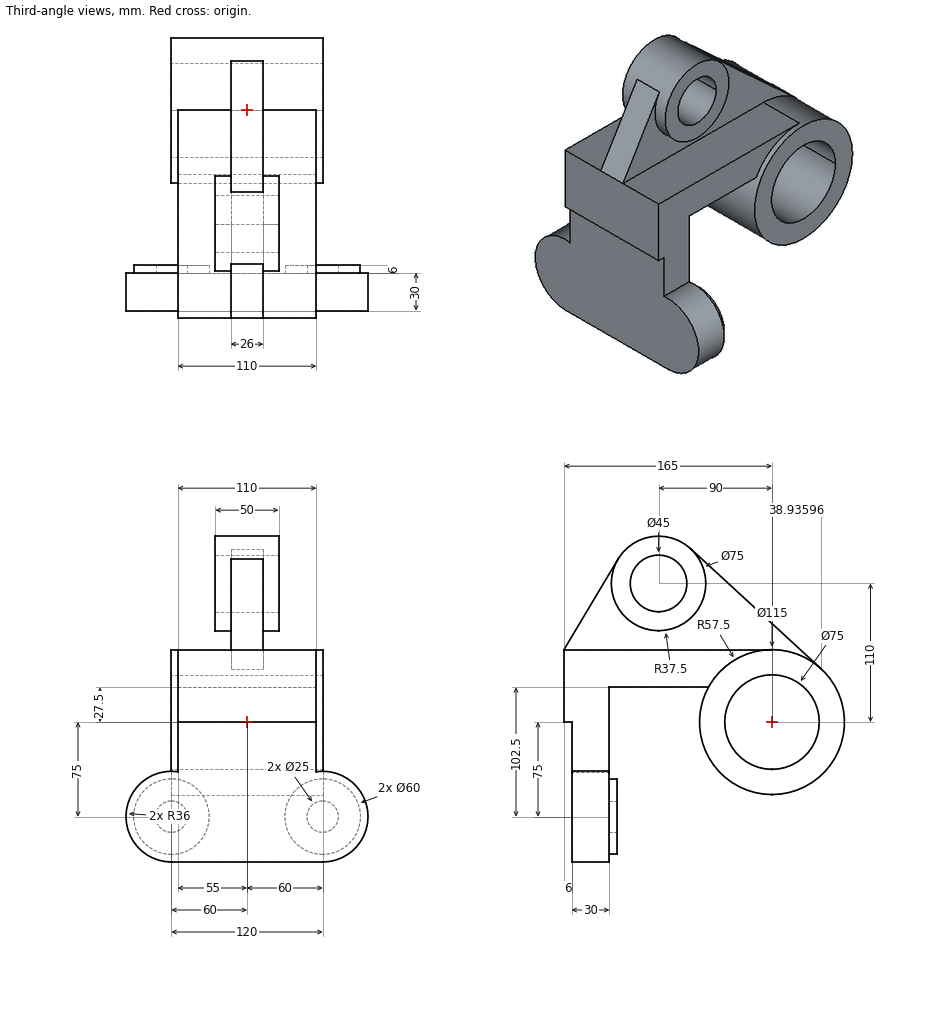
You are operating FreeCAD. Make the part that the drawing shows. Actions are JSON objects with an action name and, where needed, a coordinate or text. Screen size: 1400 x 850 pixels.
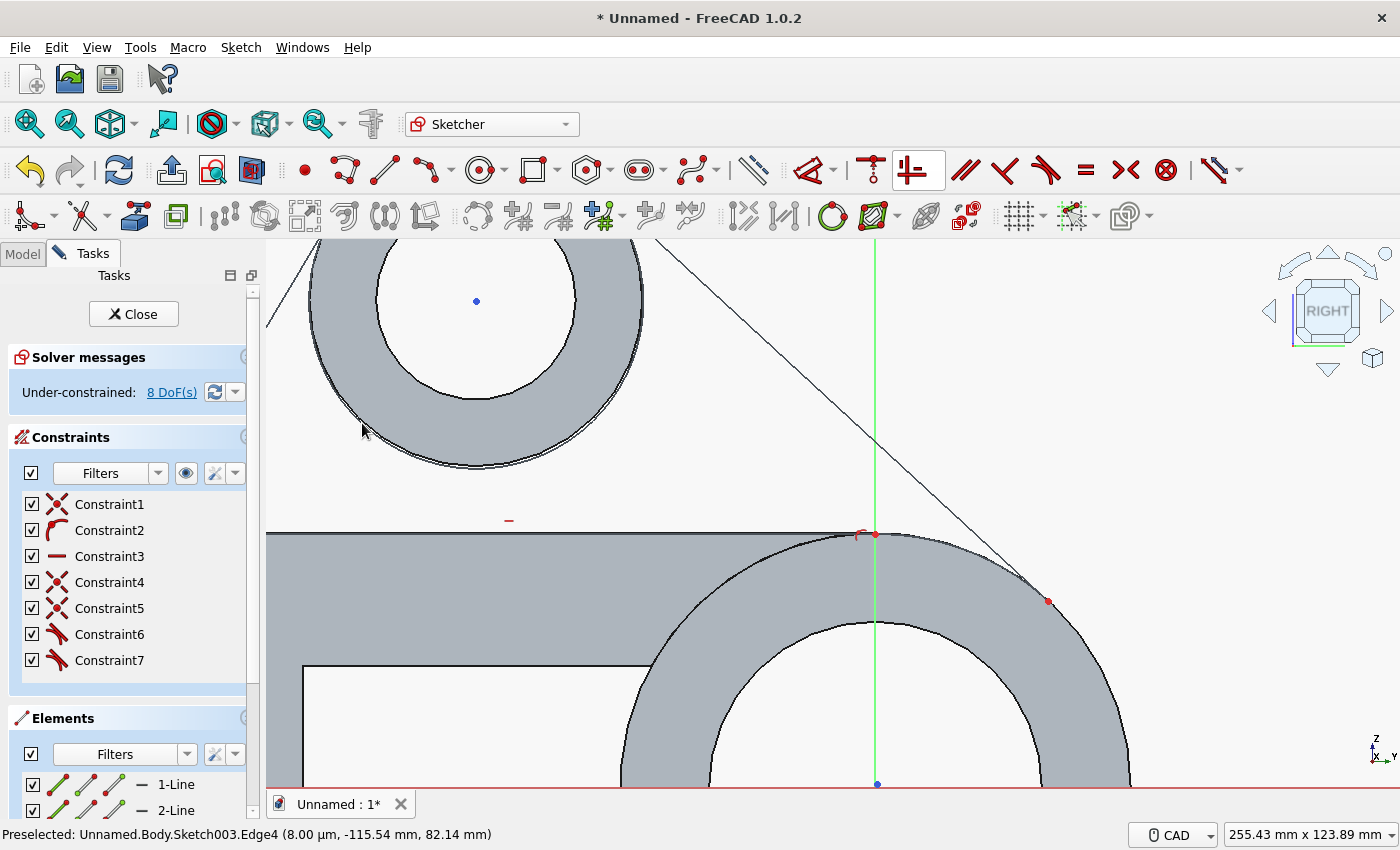
{"action": "scroll", "coordinate": [970, 552], "scroll_direction": "down", "scroll_amount": 3}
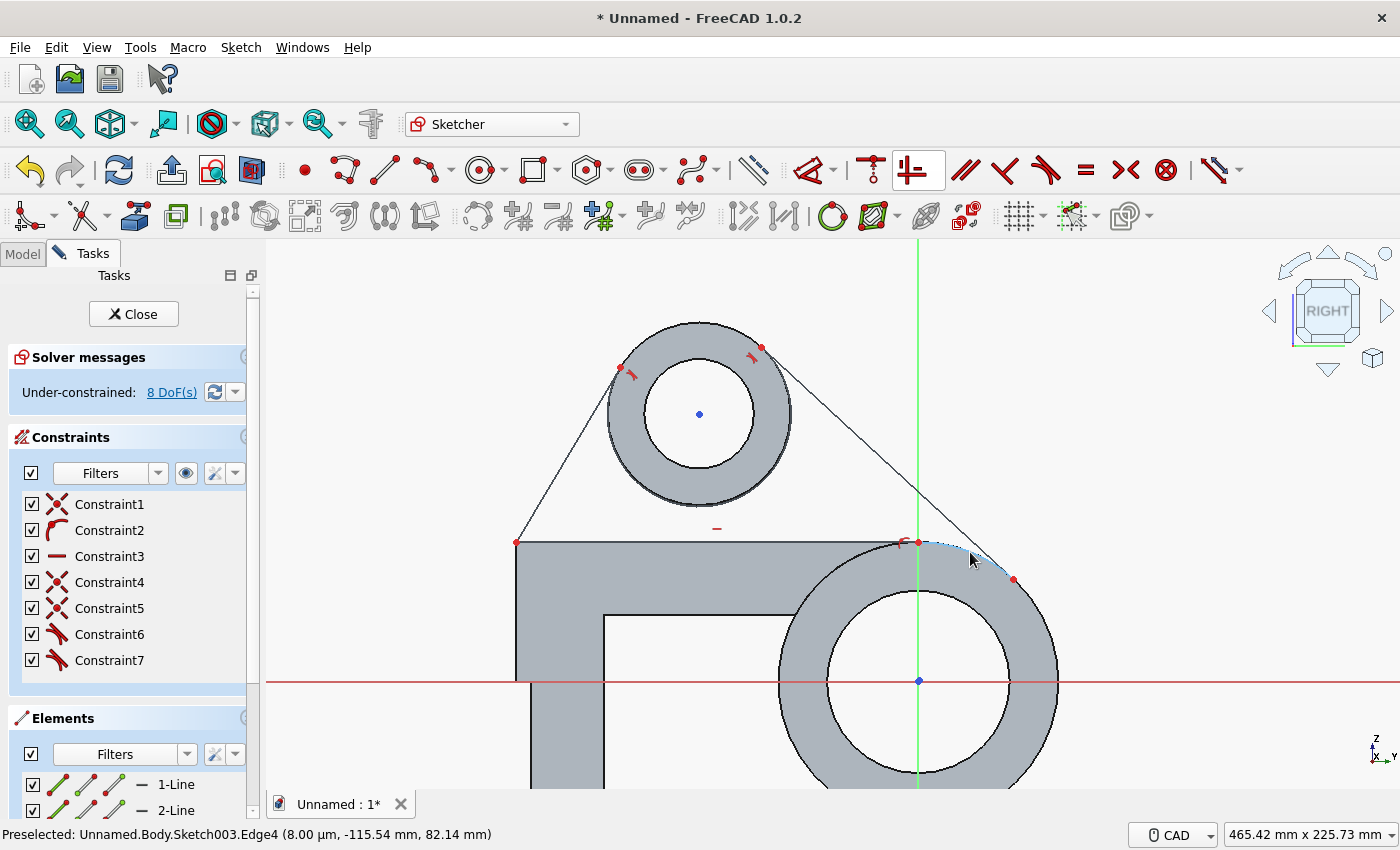
{"action": "left_click_drag", "start_coordinate": [908, 670], "coordinate": [930, 692]}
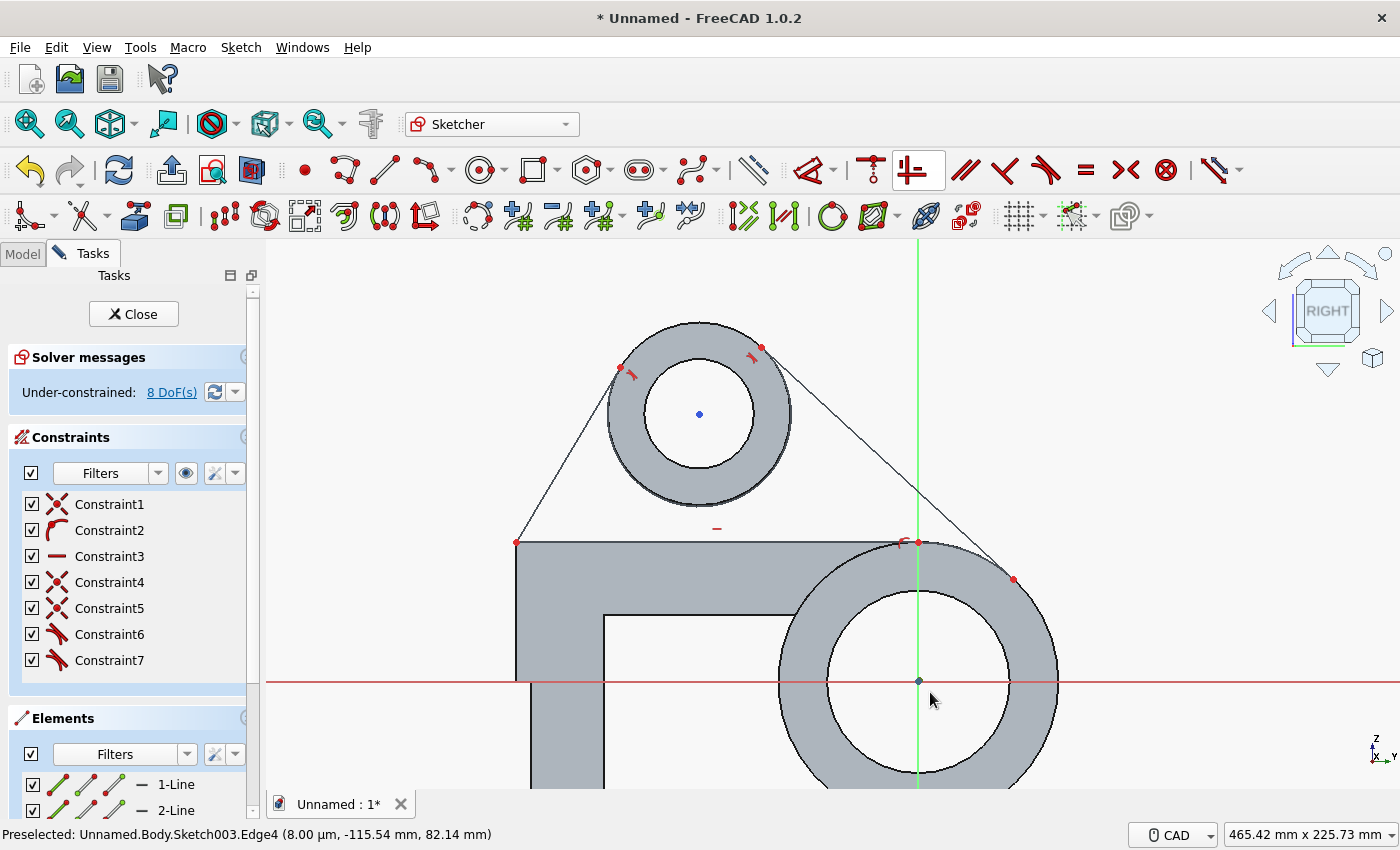
{"action": "left_click", "coordinate": [872, 170]}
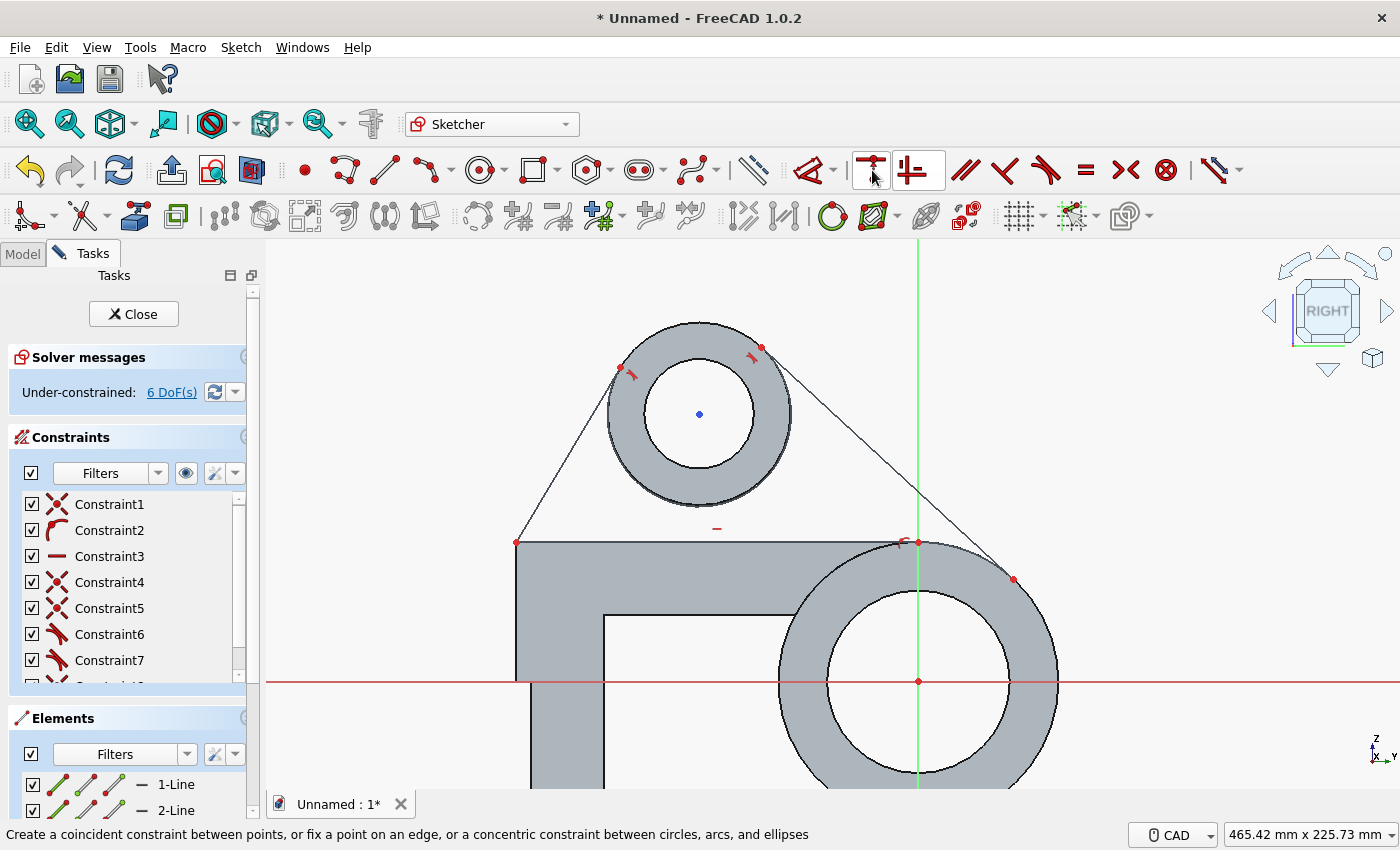
{"action": "left_click", "coordinate": [808, 170]}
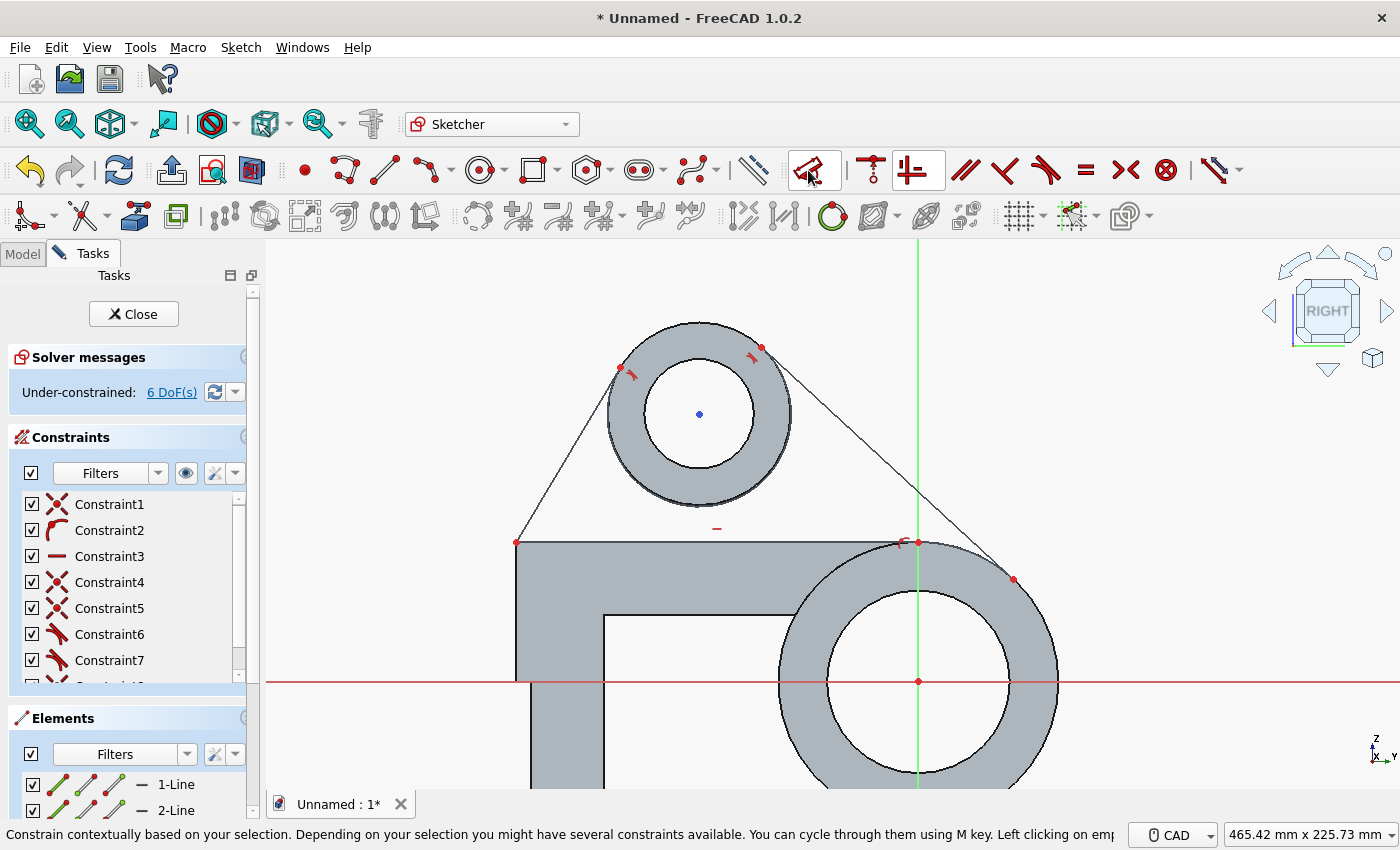
{"action": "left_click", "coordinate": [636, 482]}
{"action": "left_click", "coordinate": [614, 505]}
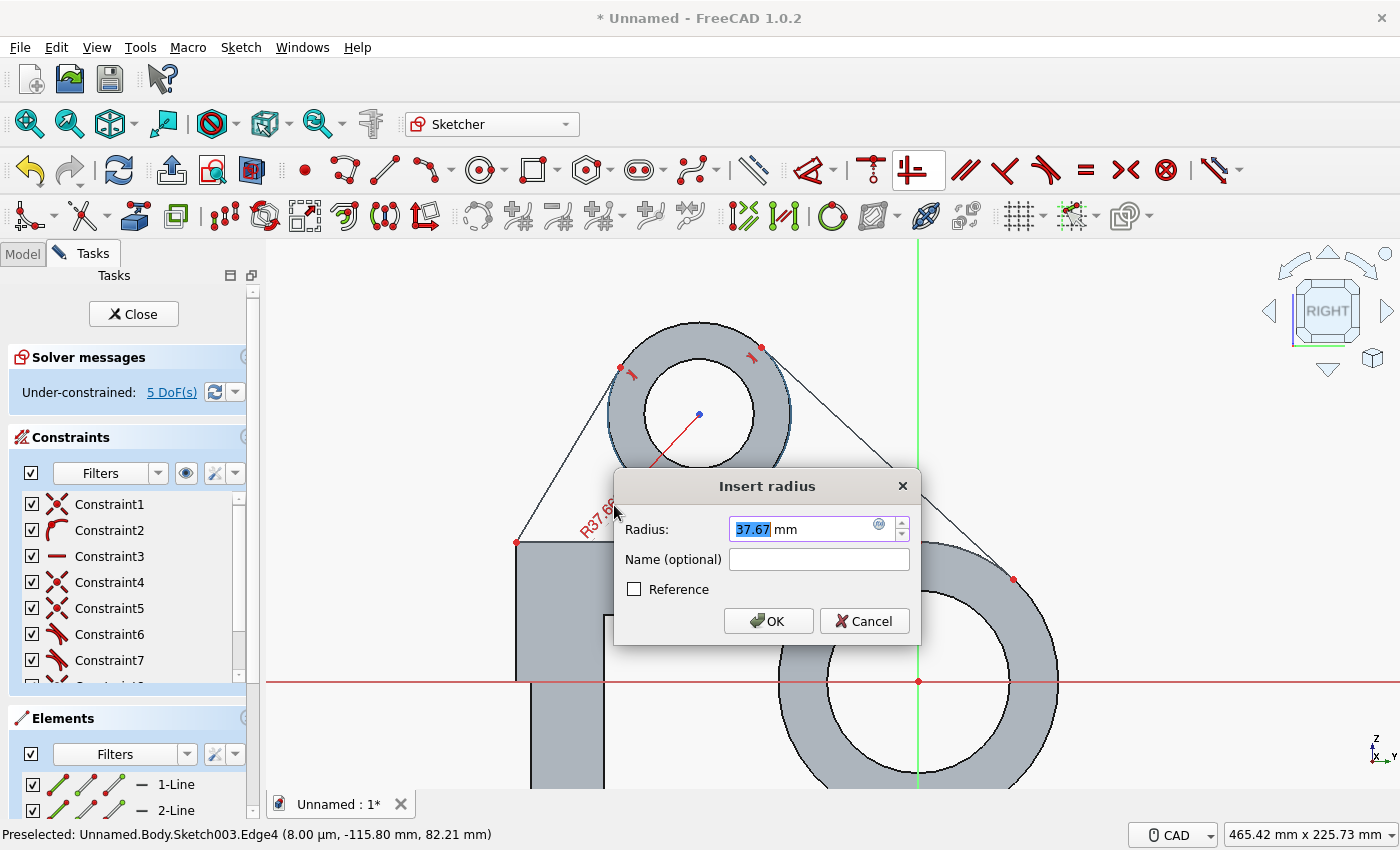
{"action": "type", "text": "37.5"}
{"action": "key", "text": "Return"}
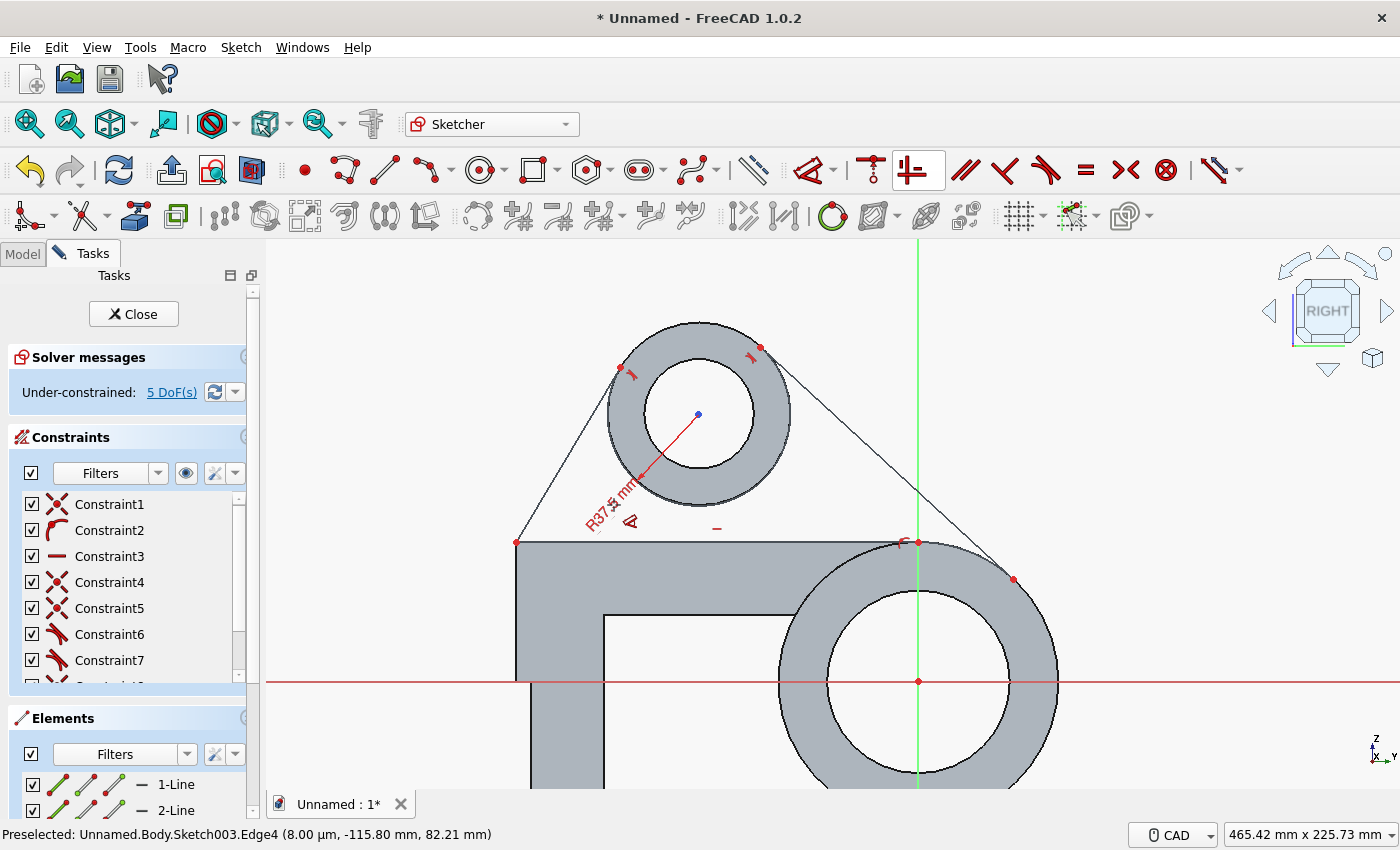
{"action": "left_click", "coordinate": [949, 546]}
{"action": "left_click", "coordinate": [1032, 553]}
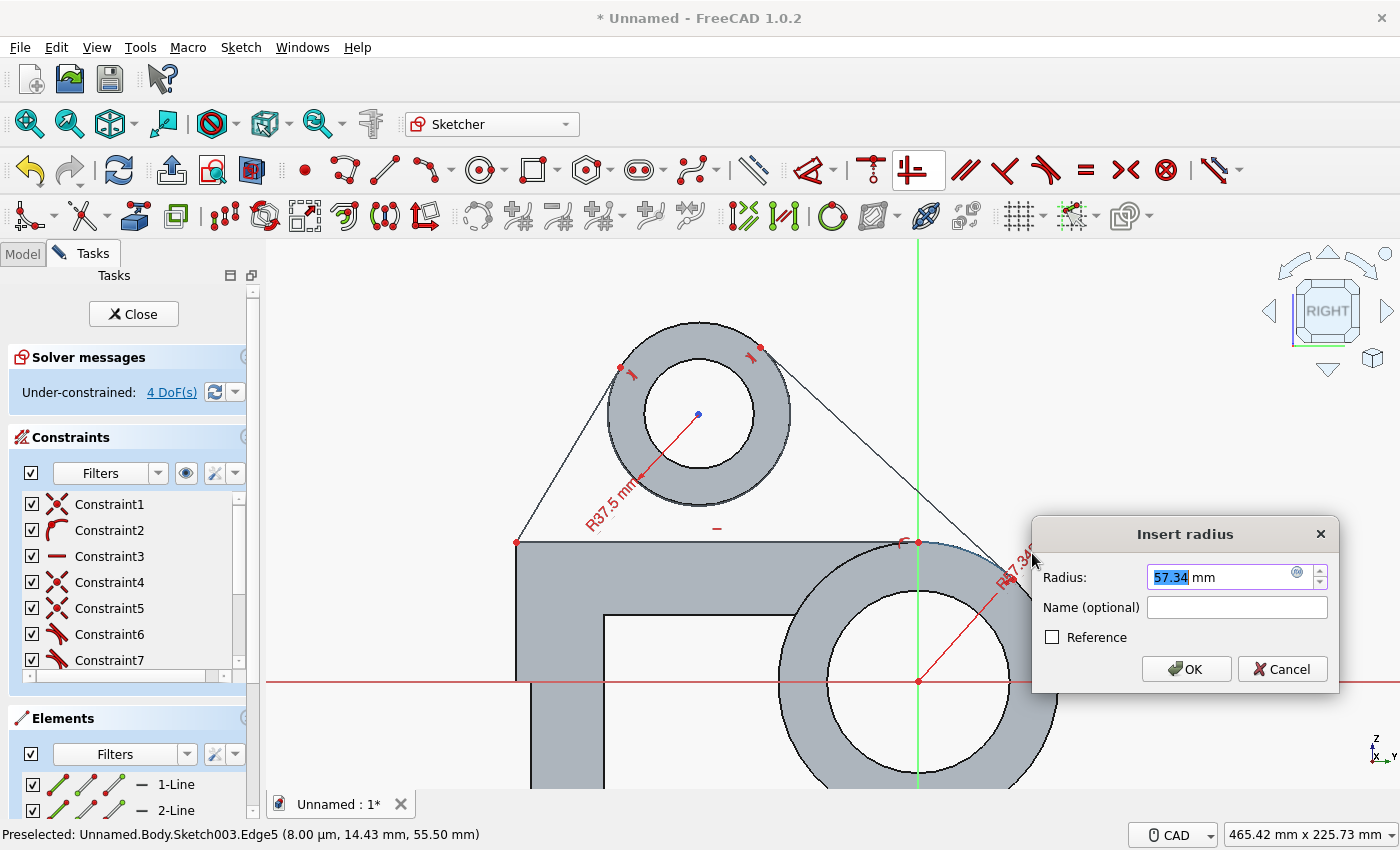
{"action": "type", "text": "57.5"}
{"action": "key", "text": "Return"}